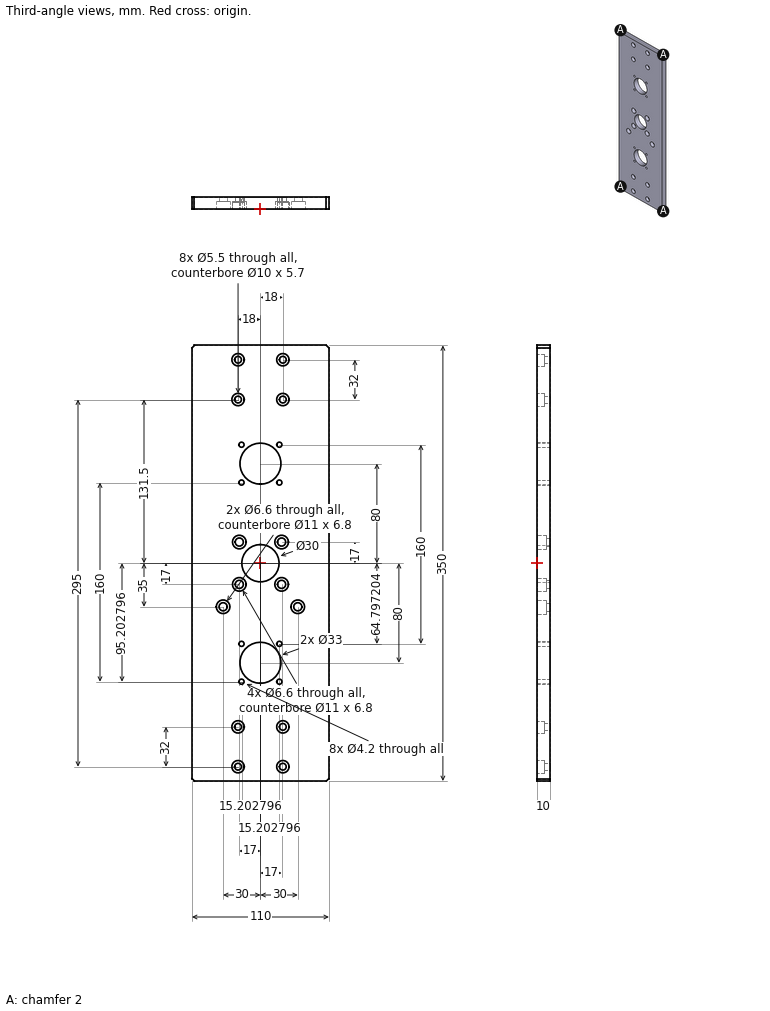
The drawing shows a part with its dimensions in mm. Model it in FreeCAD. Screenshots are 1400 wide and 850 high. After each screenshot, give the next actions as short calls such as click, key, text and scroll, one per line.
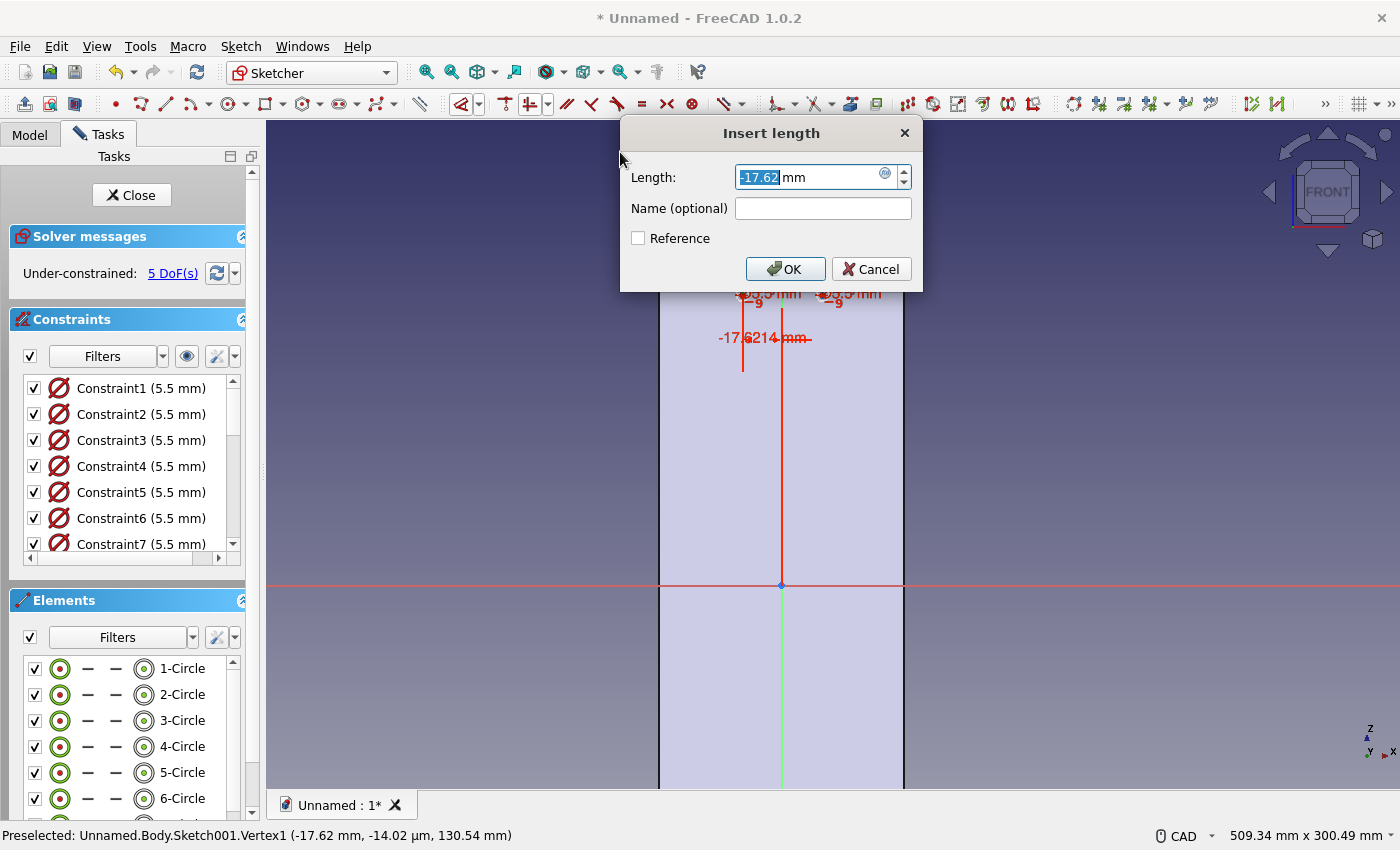
text(-18)
key(Return)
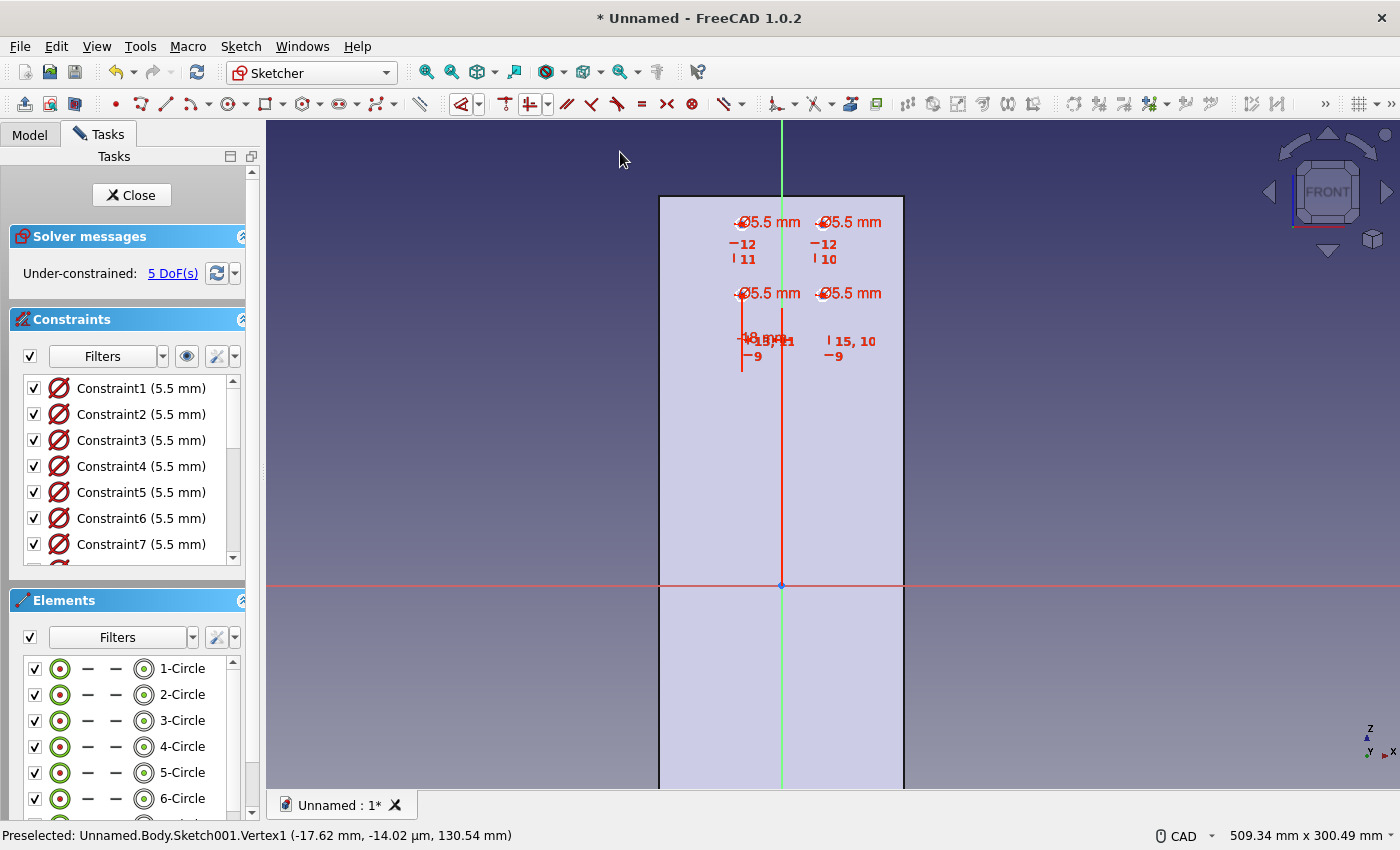
click(823, 295)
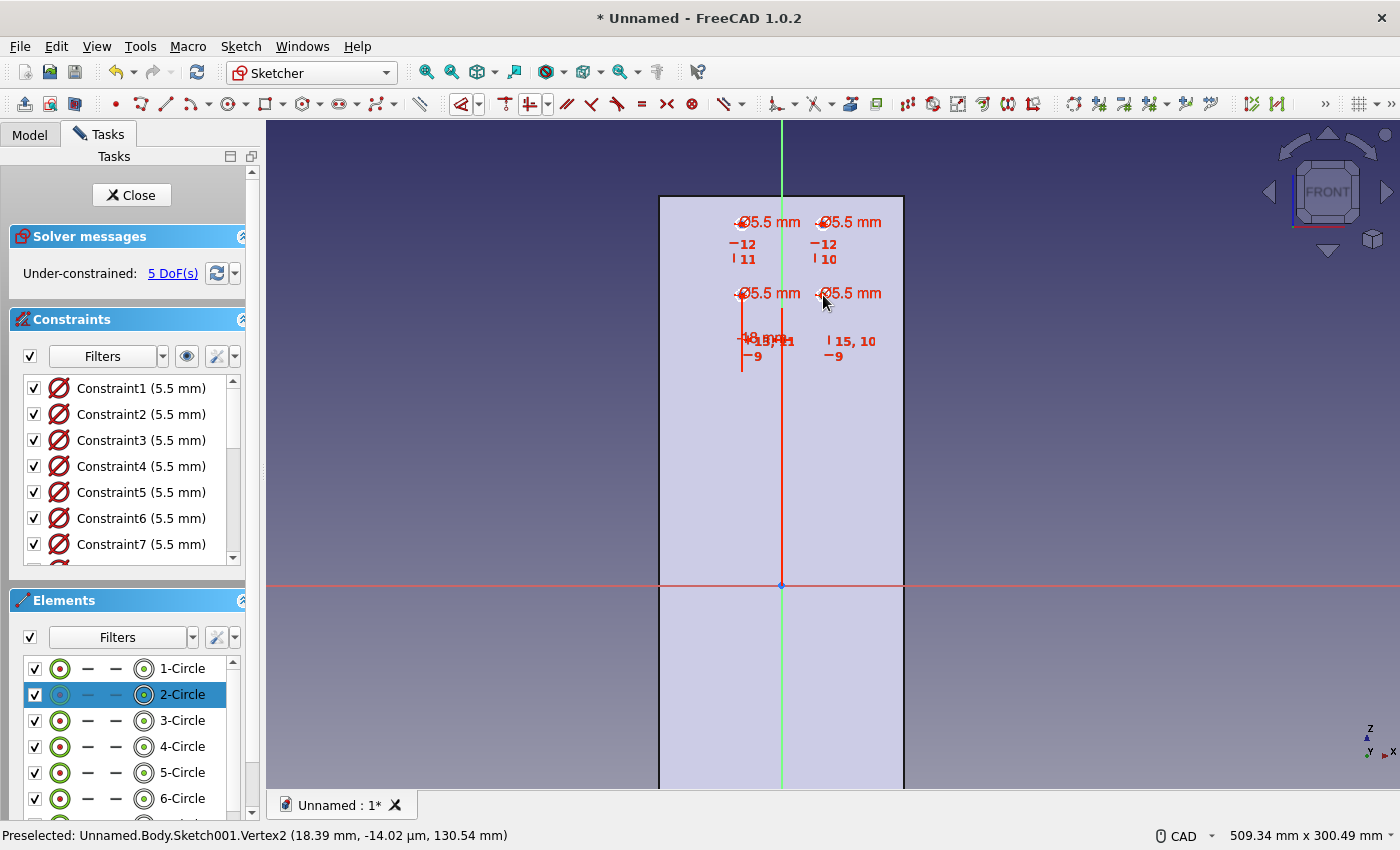
key(l)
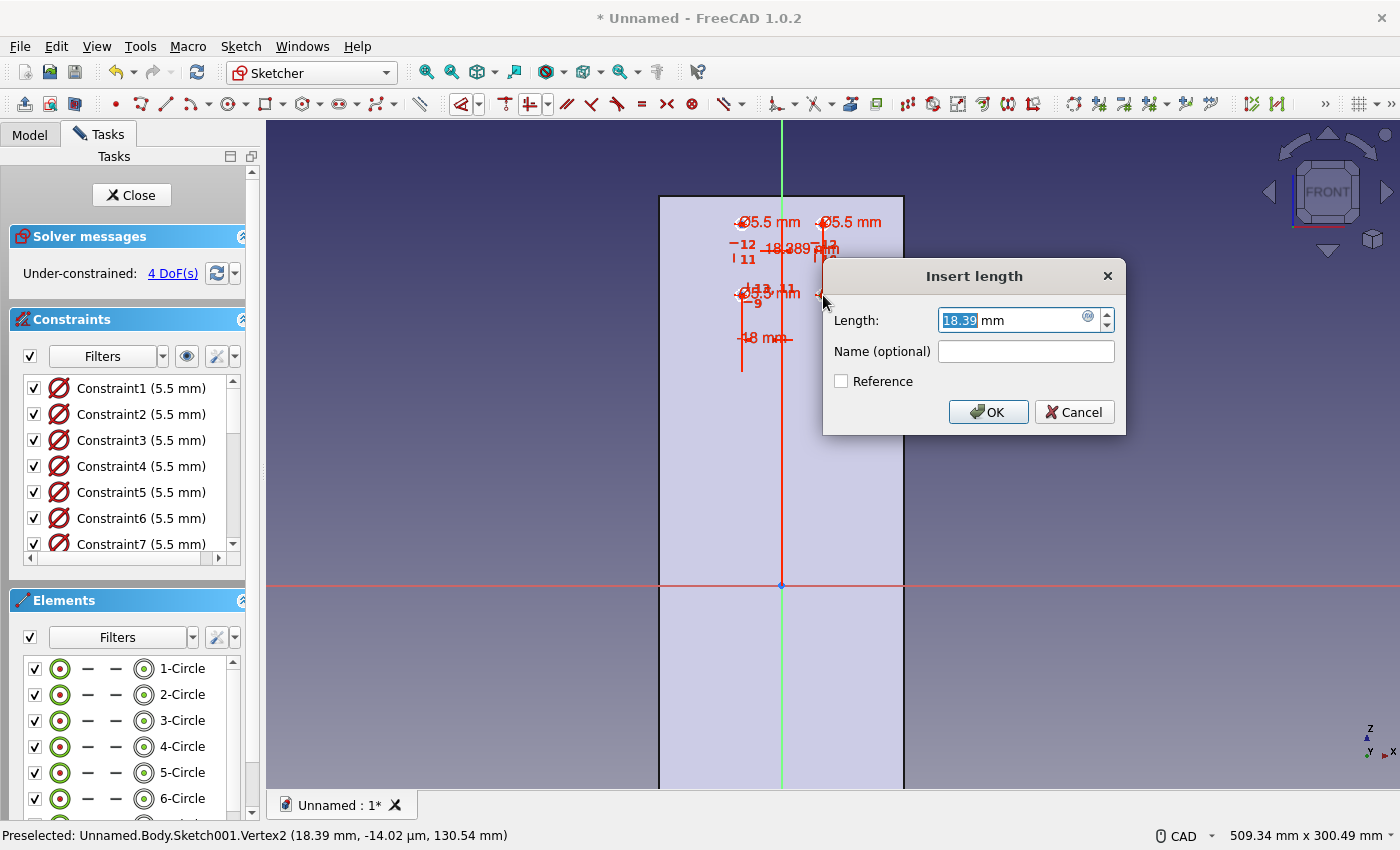
text(18)
key(Return)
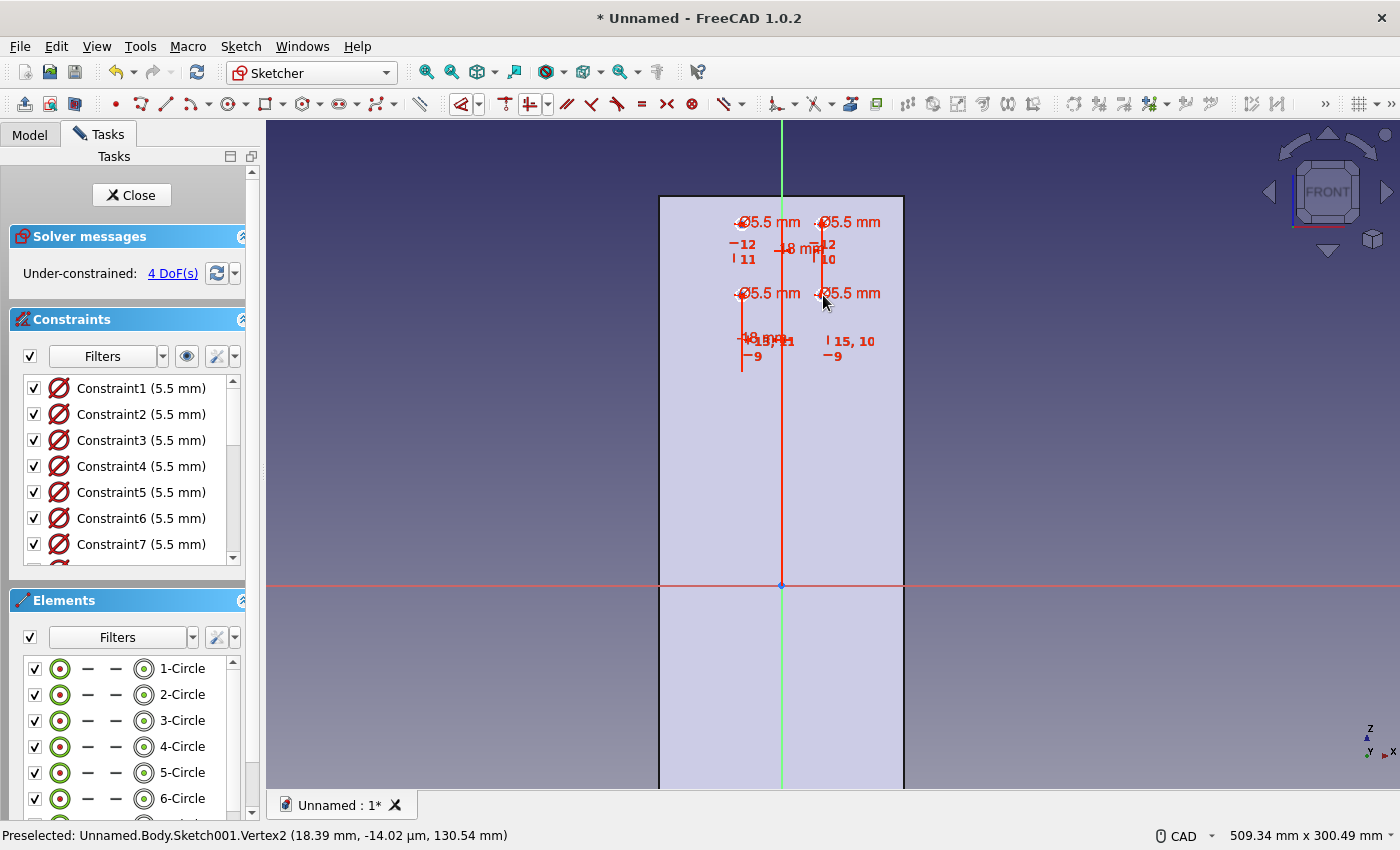
click(822, 295)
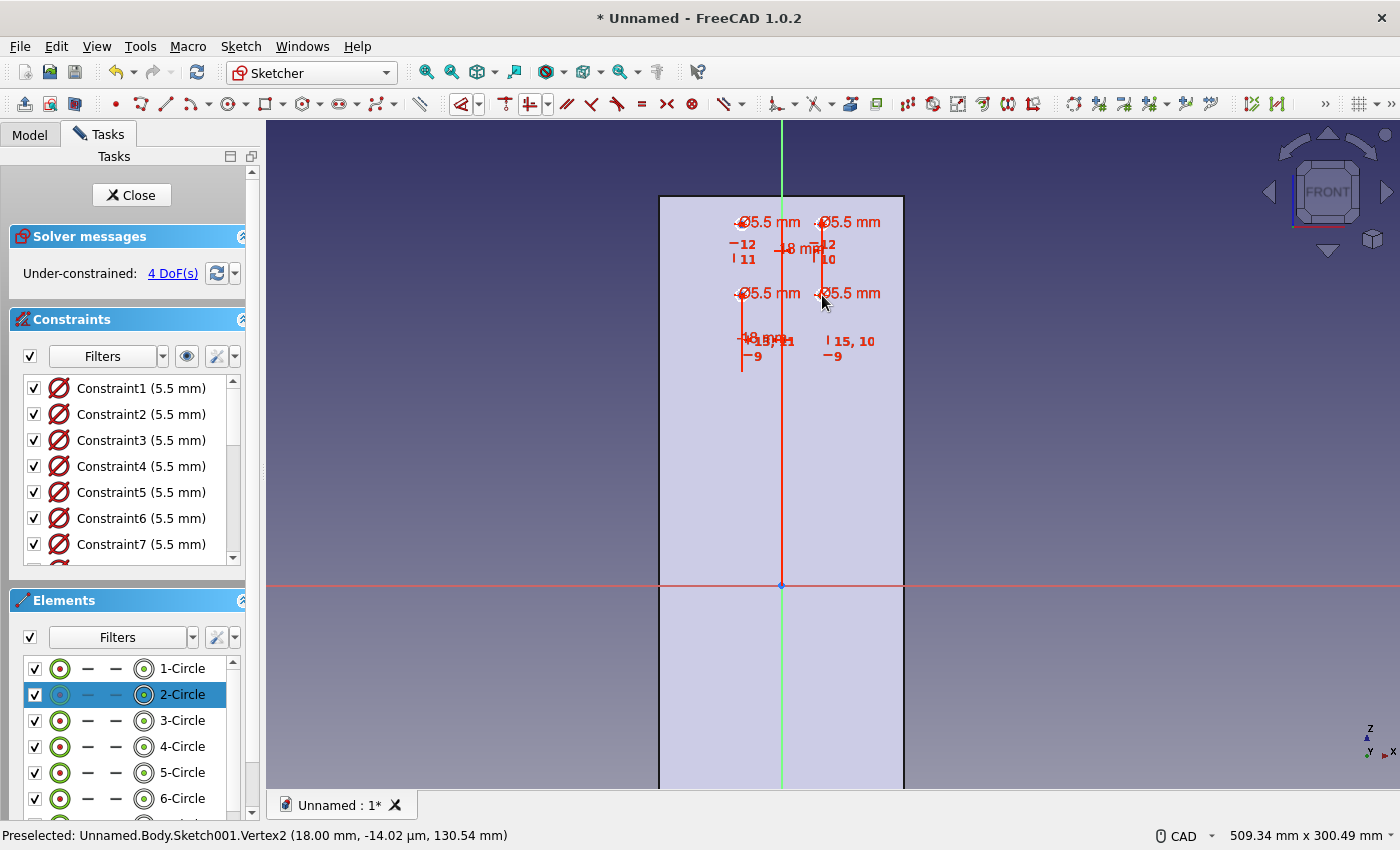
click(822, 224)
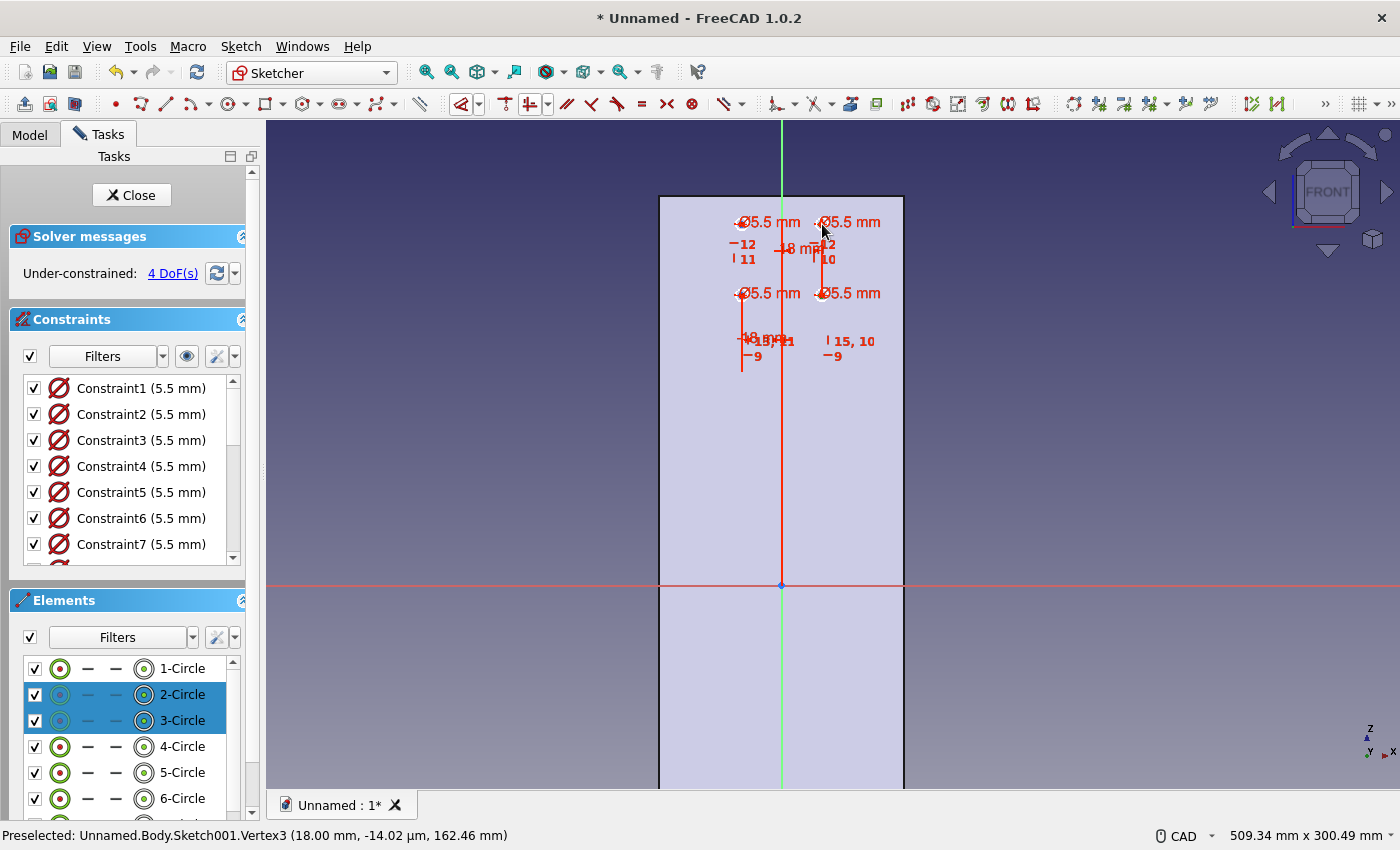
key(i)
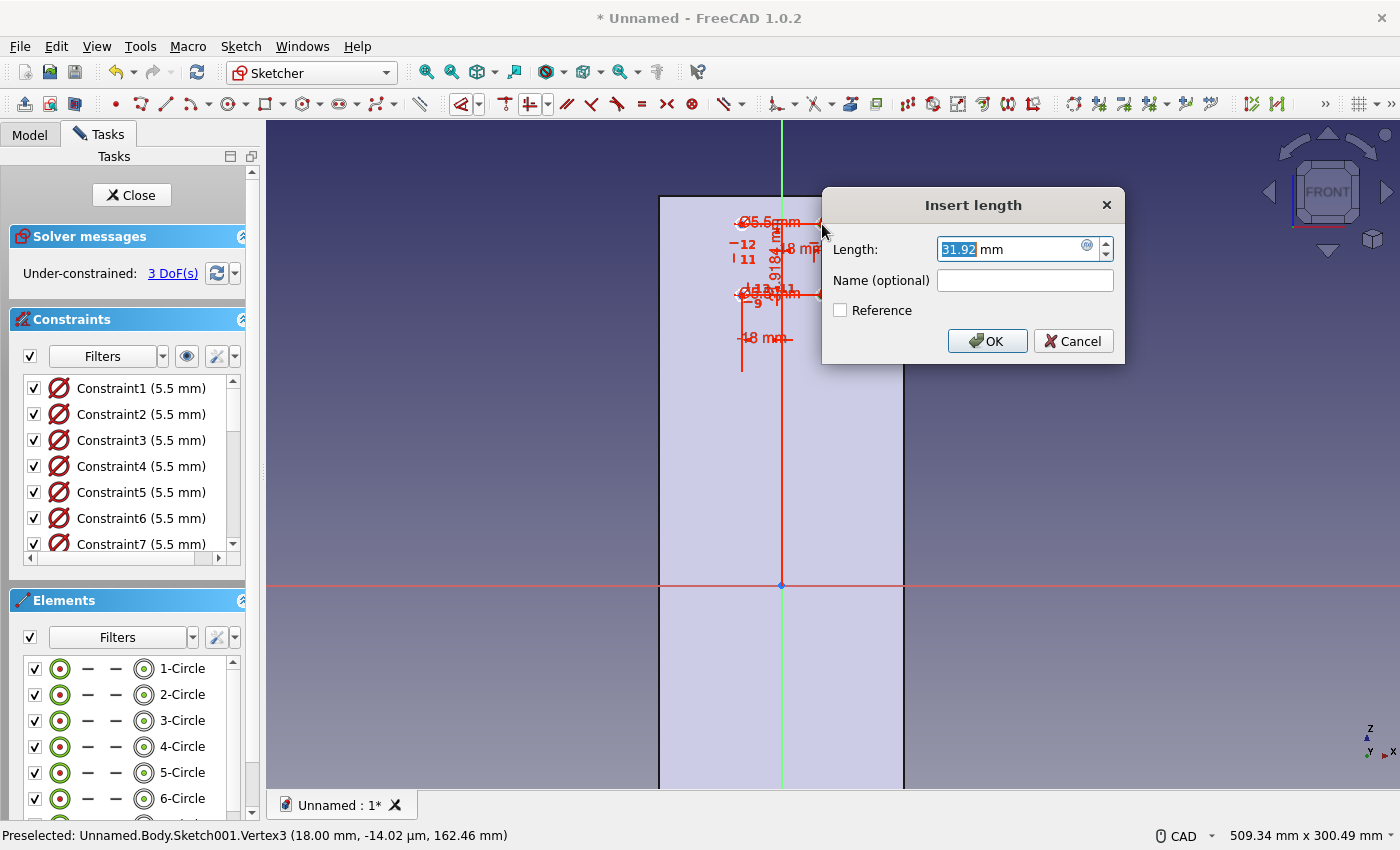
text(32)
key(Return)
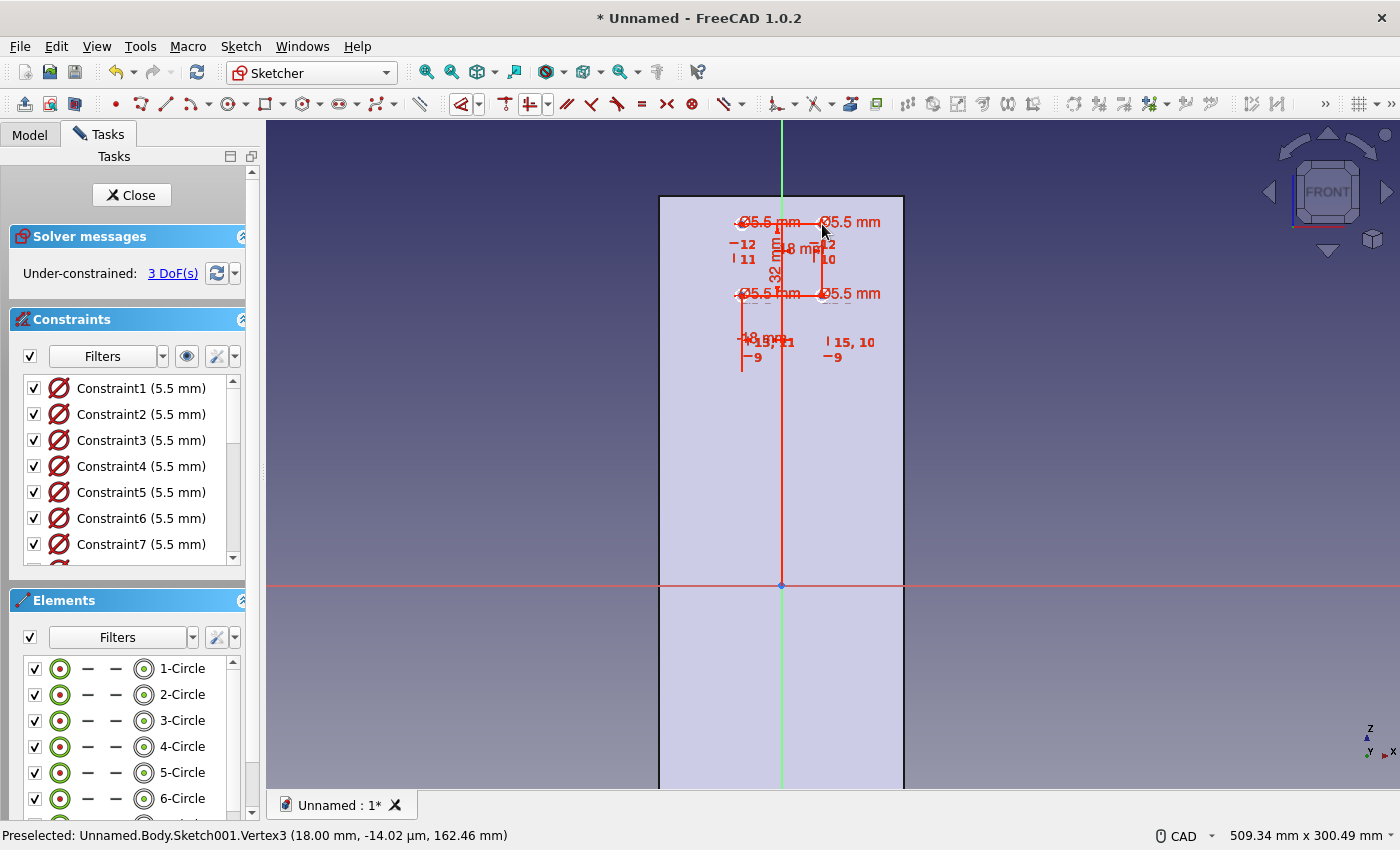
scroll(743, 295, down, 3)